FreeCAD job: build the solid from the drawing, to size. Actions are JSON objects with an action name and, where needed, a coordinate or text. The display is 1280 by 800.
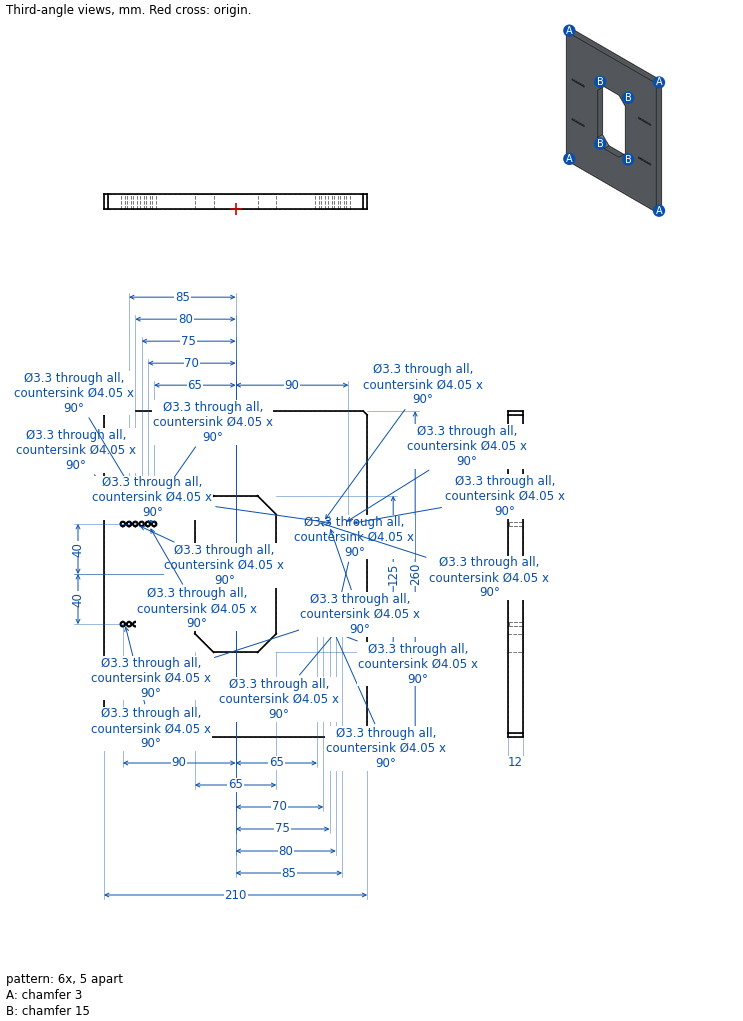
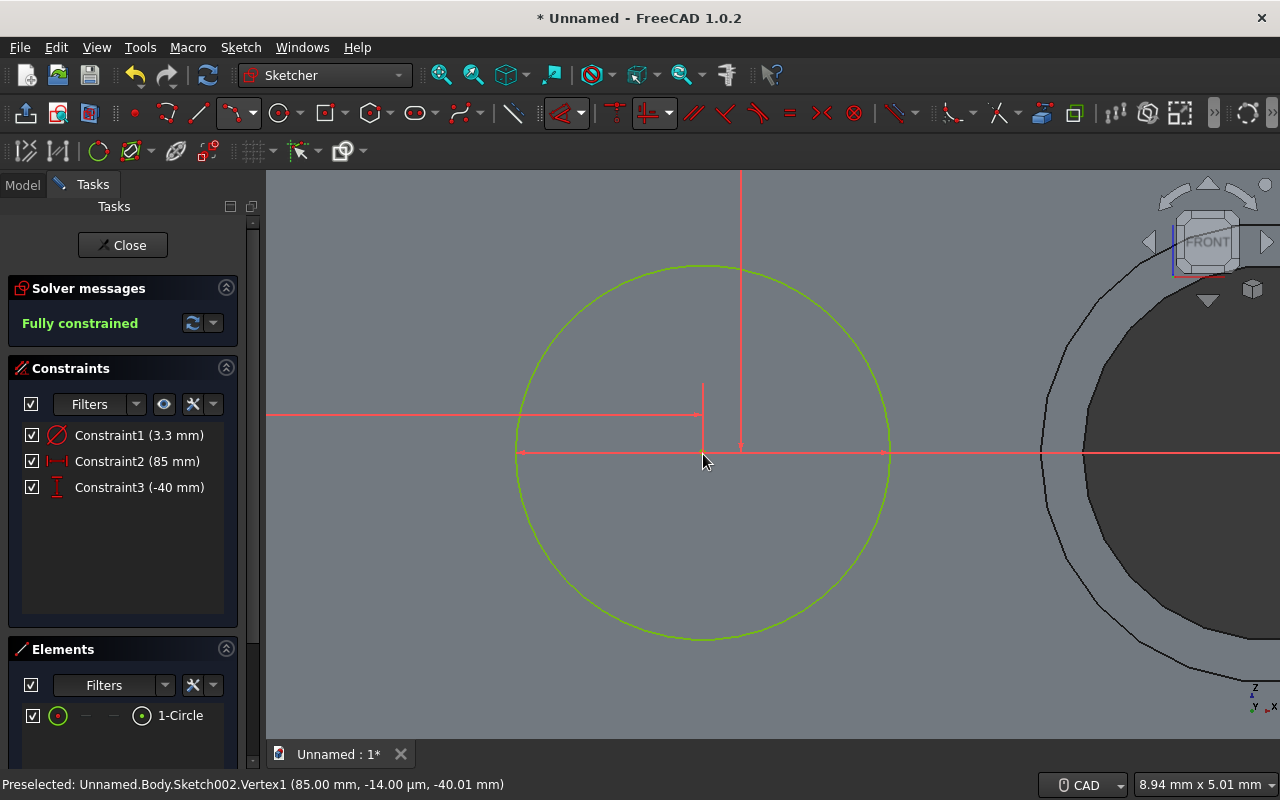
{"action": "left_click", "coordinate": [123, 245]}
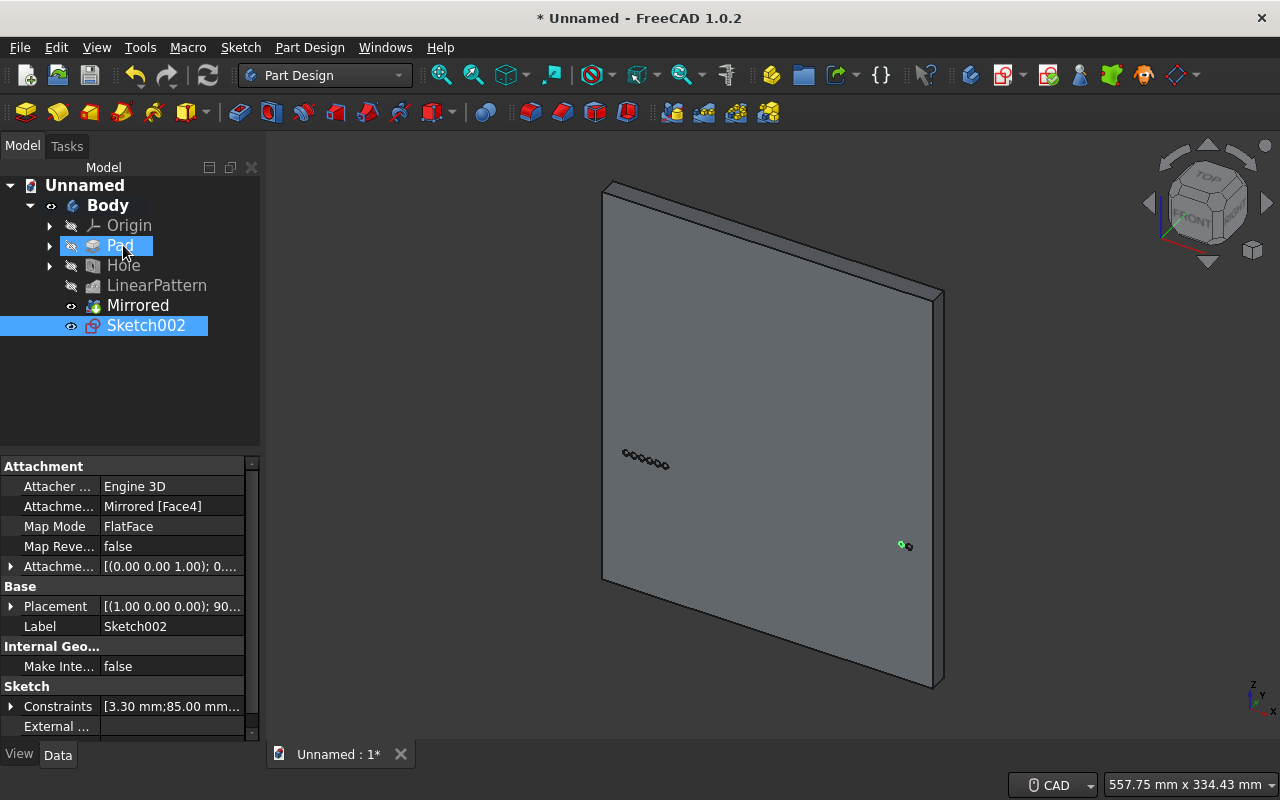
{"action": "left_click", "coordinate": [272, 112]}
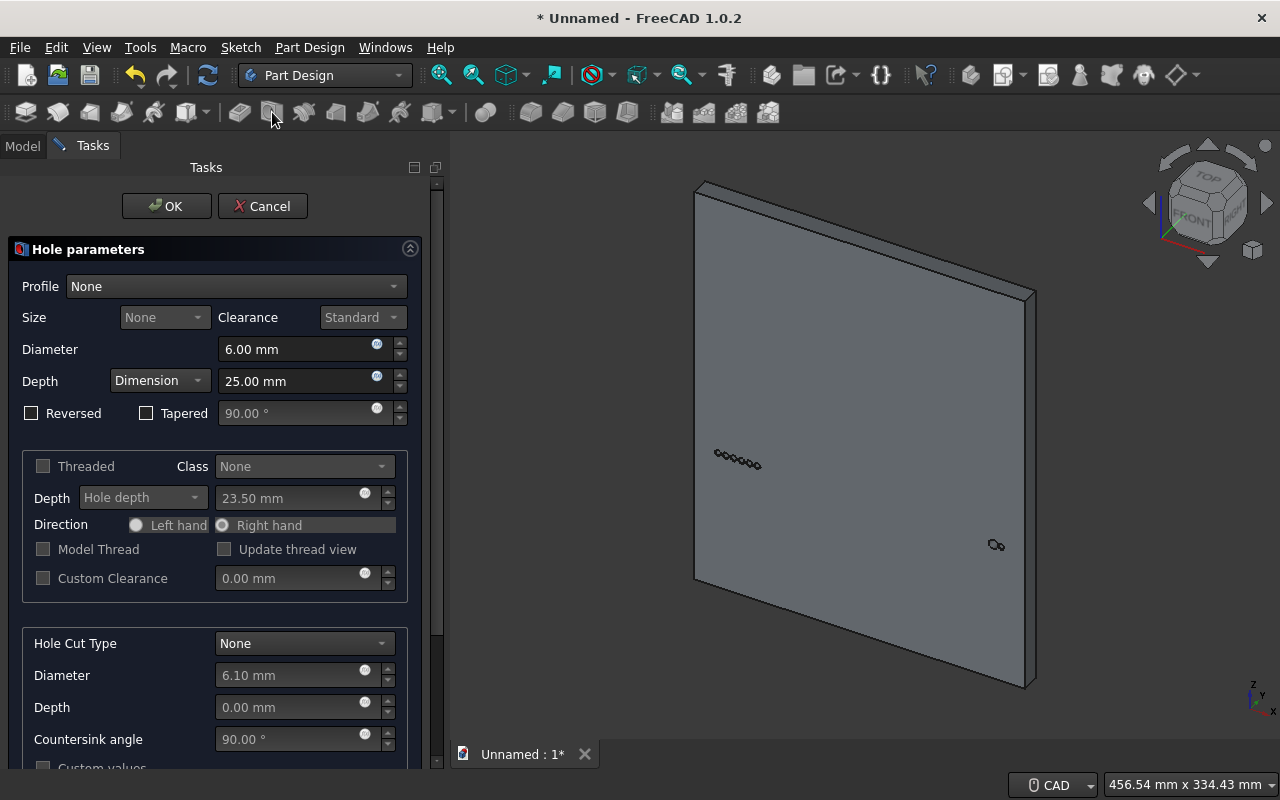
{"action": "triple_click", "coordinate": [305, 349]}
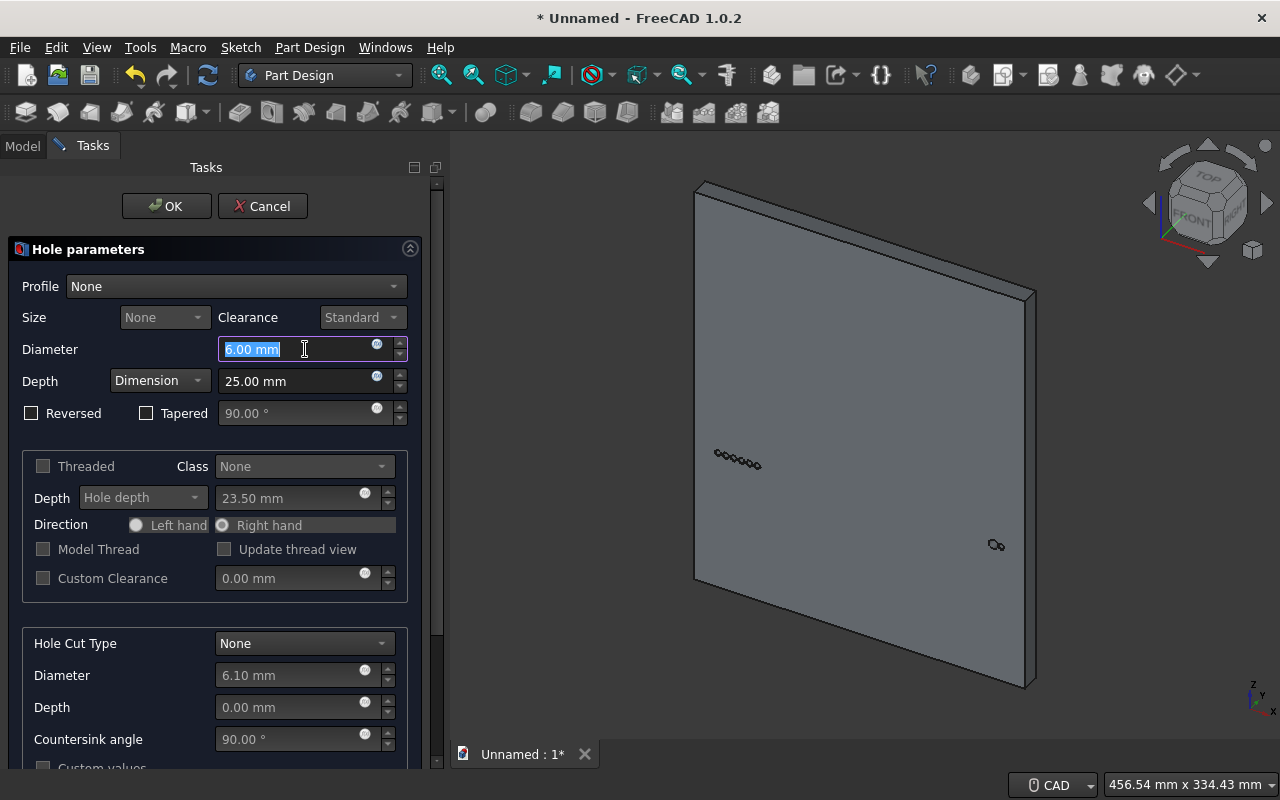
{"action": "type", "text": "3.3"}
{"action": "key", "text": "Tab"}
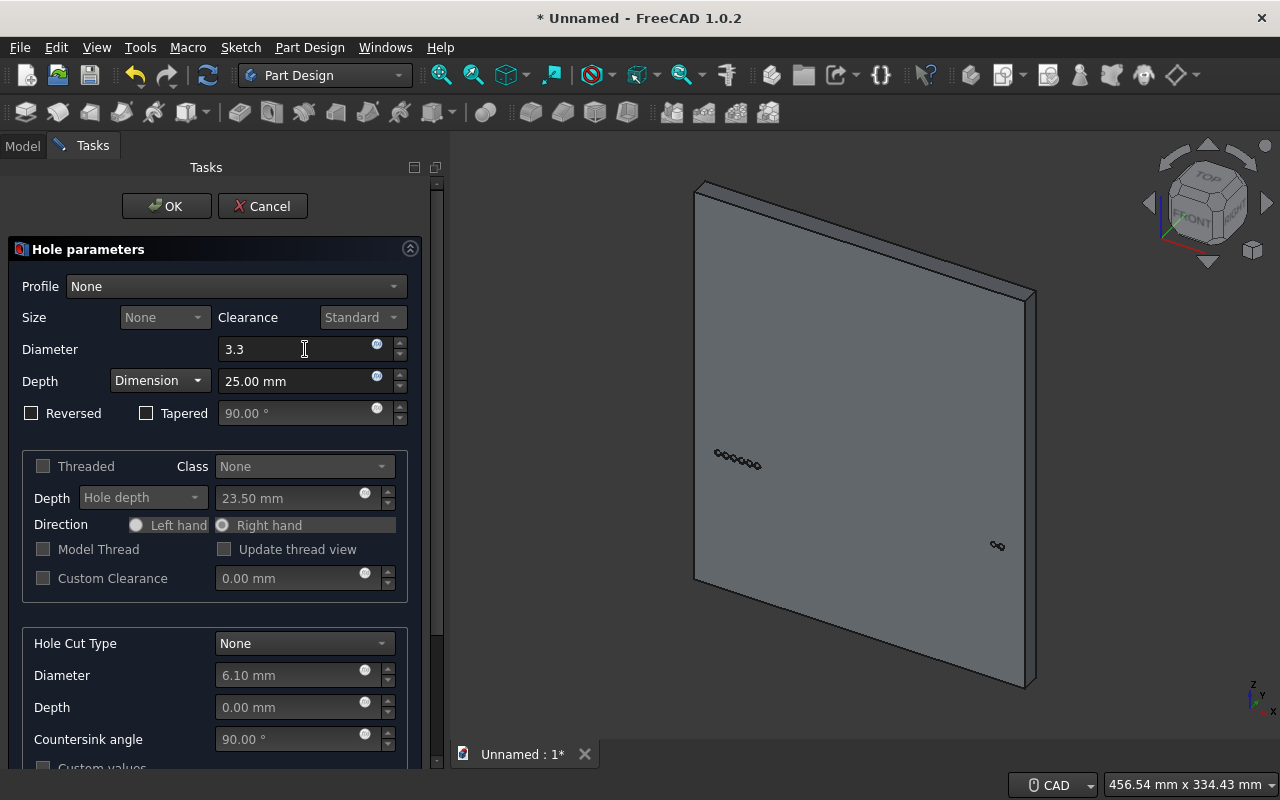
{"action": "left_click", "coordinate": [161, 380]}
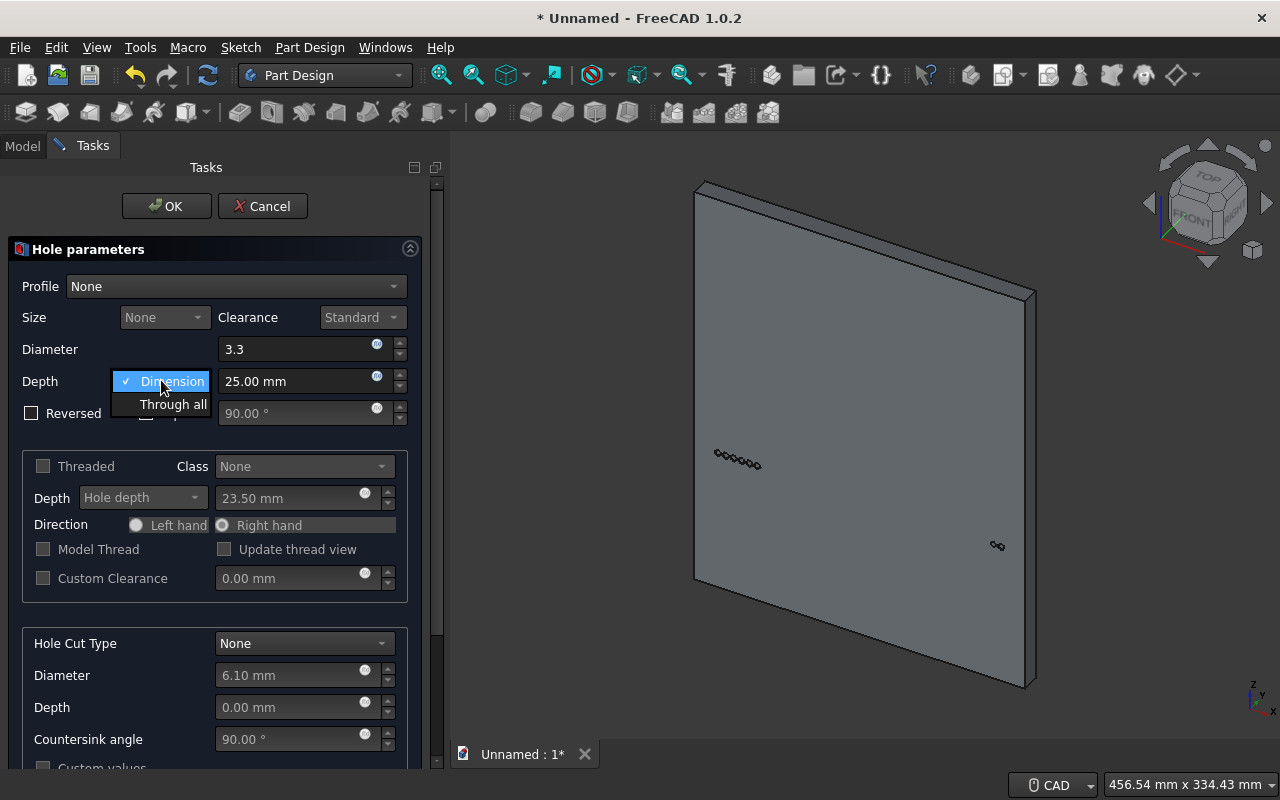
{"action": "left_click", "coordinate": [160, 404]}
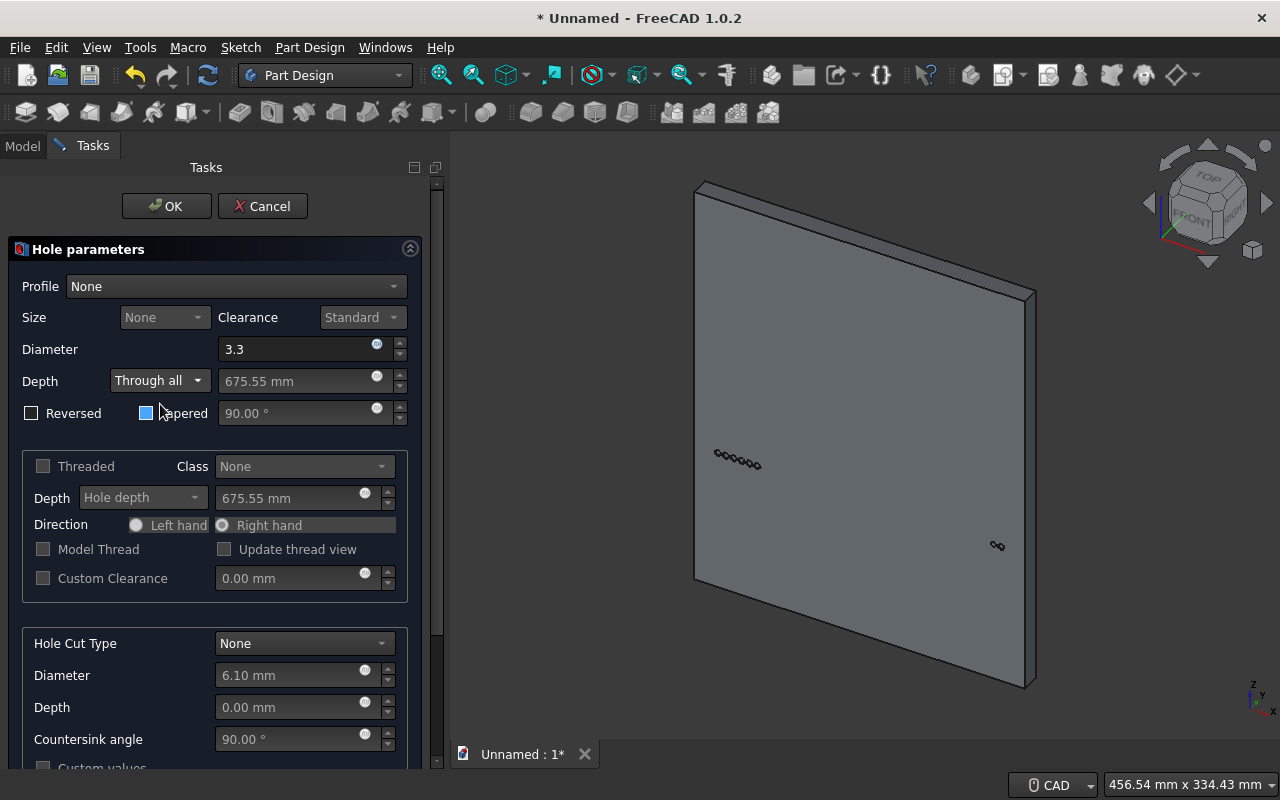
{"action": "left_click", "coordinate": [306, 644]}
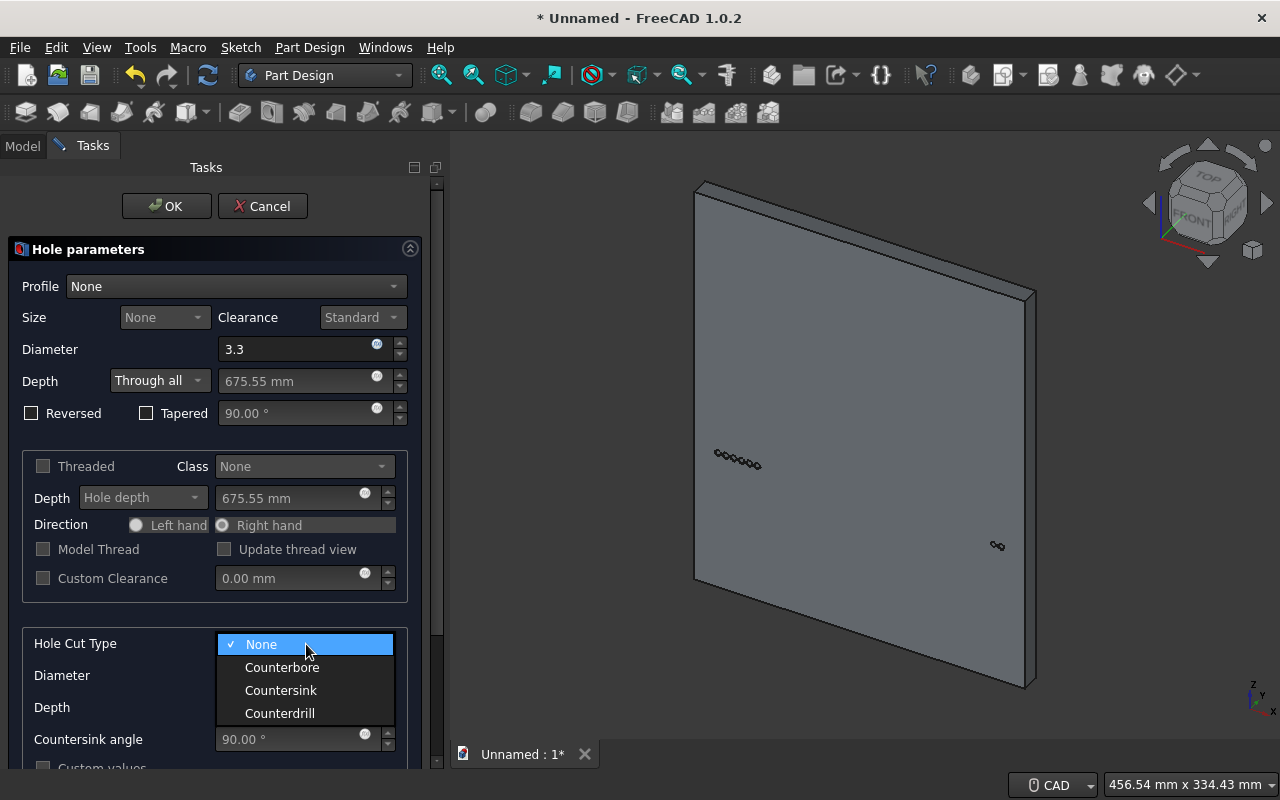
{"action": "left_click", "coordinate": [304, 690]}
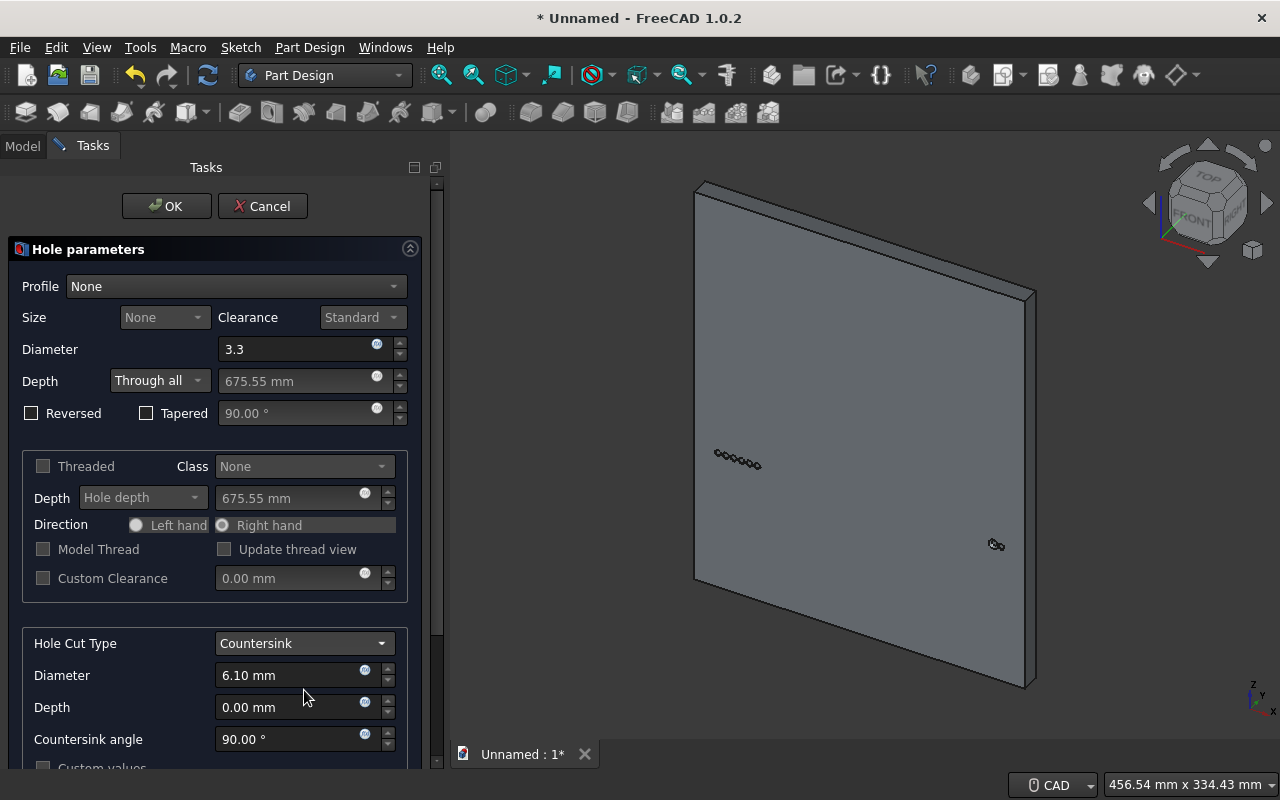
{"action": "triple_click", "coordinate": [298, 675]}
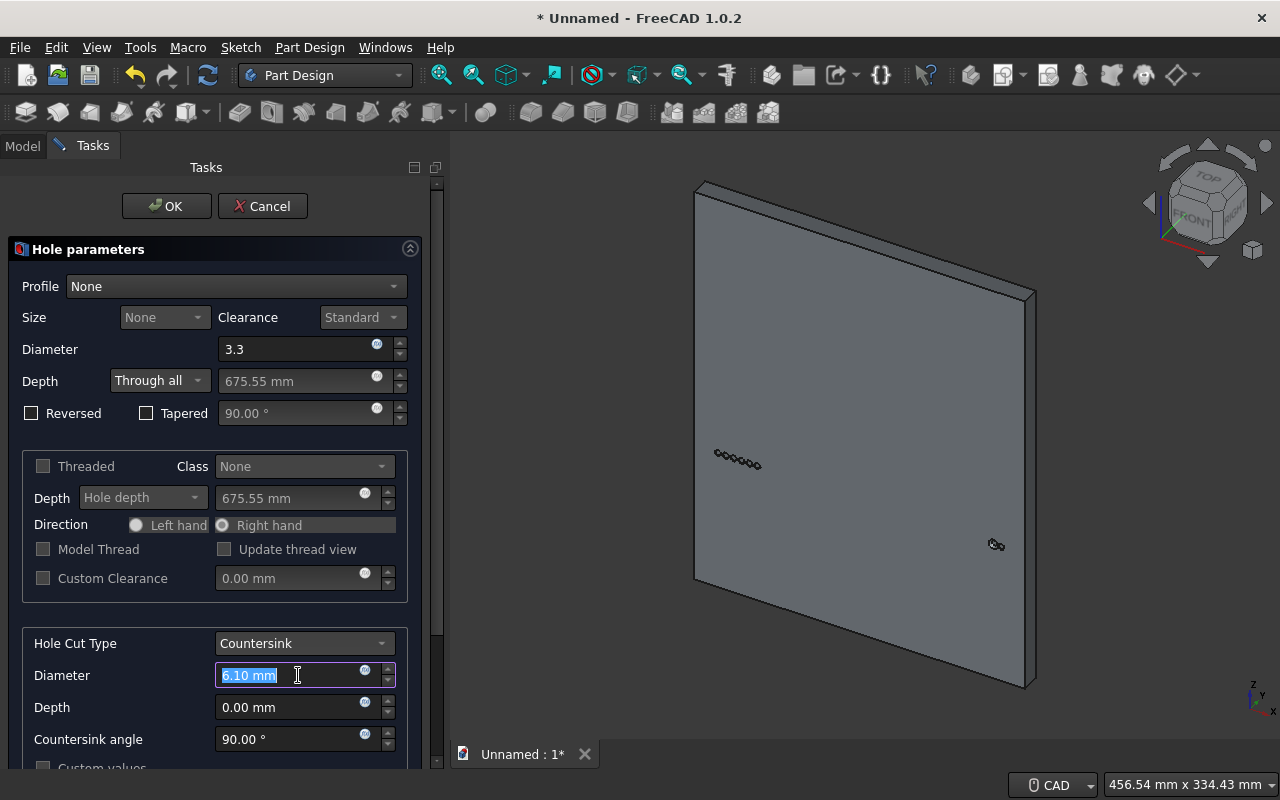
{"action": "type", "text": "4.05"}
{"action": "key", "text": "Tab"}